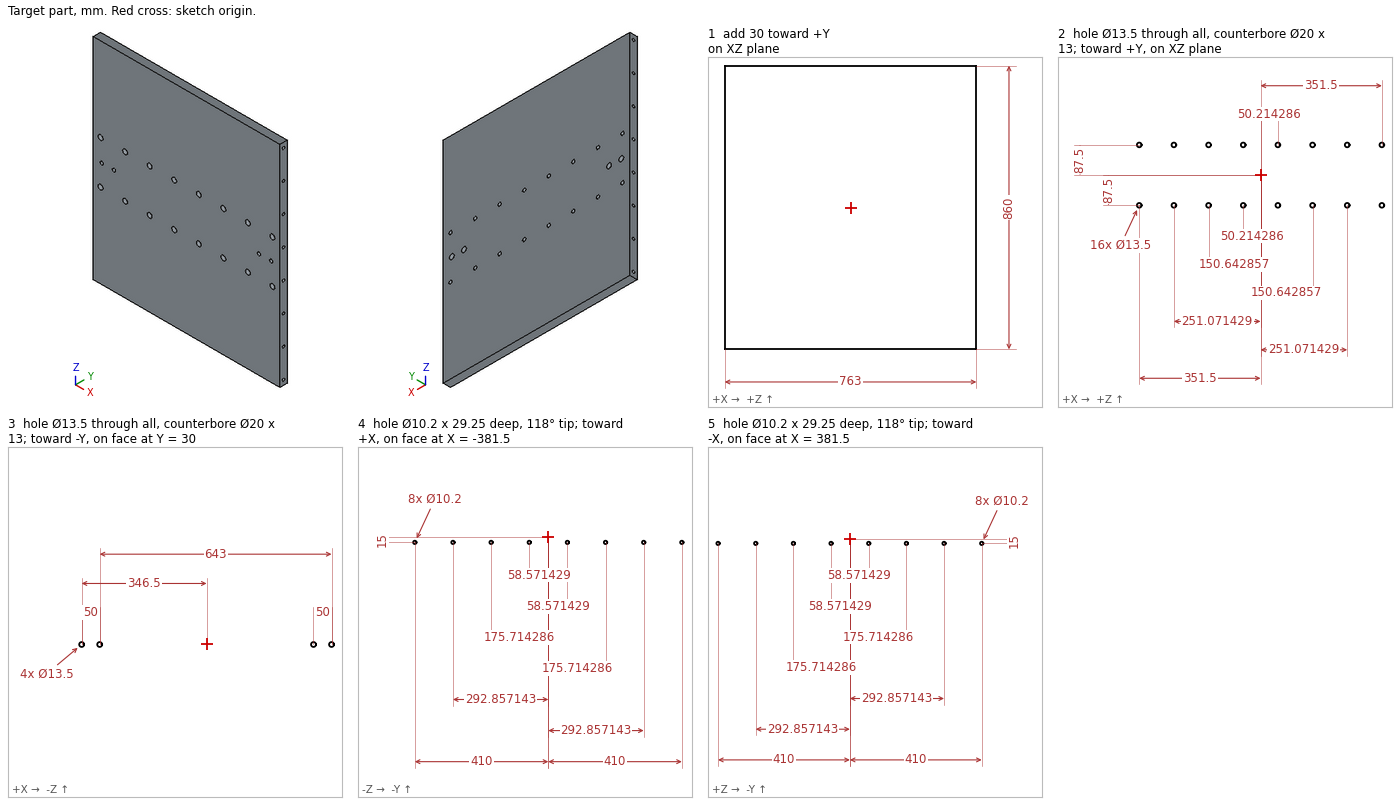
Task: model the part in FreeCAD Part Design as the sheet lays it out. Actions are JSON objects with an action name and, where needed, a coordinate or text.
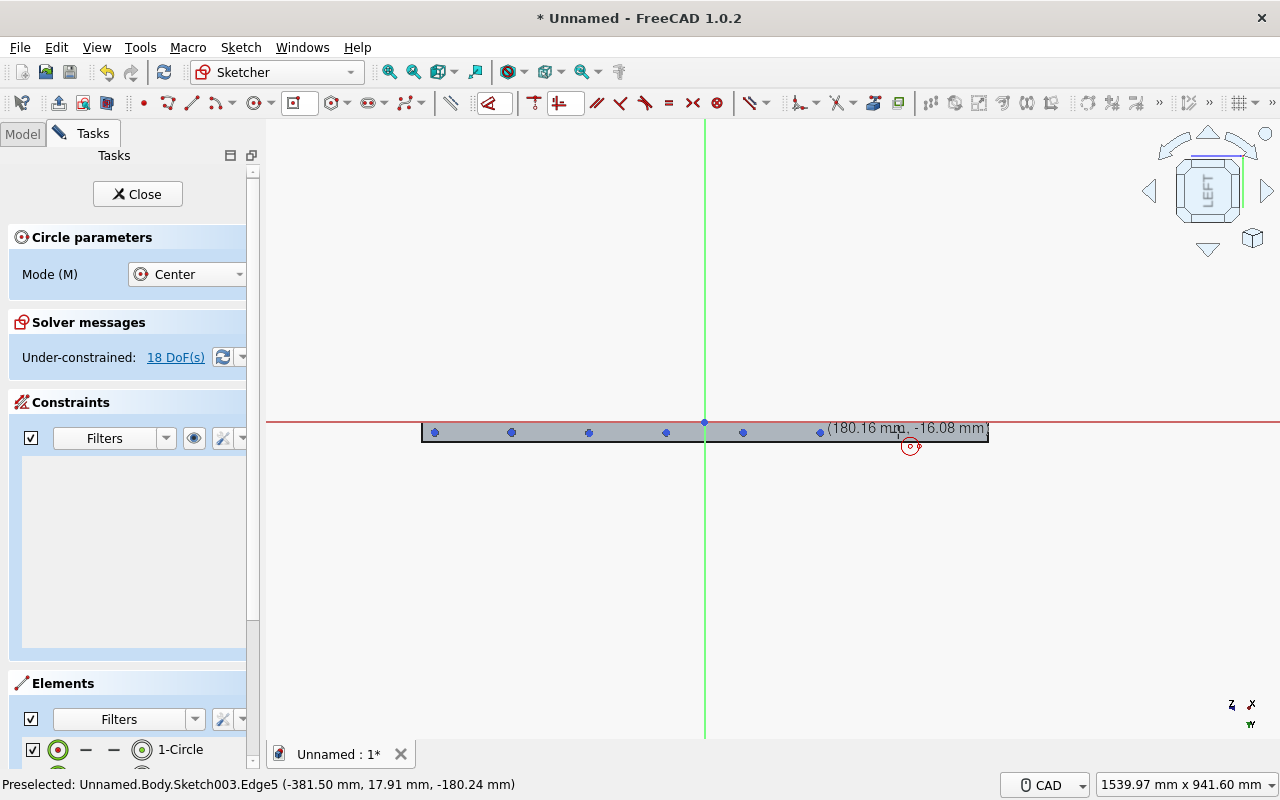
{"action": "scroll", "coordinate": [898, 432], "scroll_direction": "up", "scroll_amount": 3}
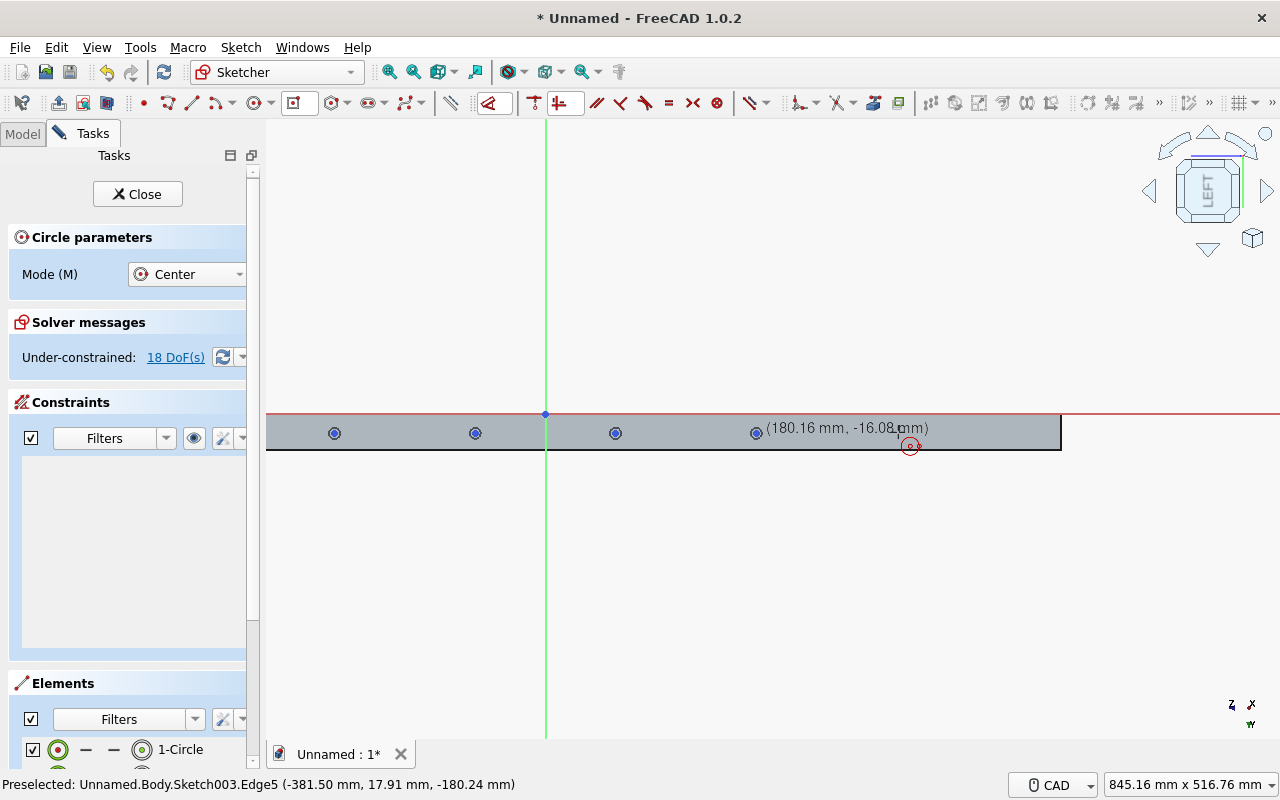
{"action": "left_click", "coordinate": [897, 432]}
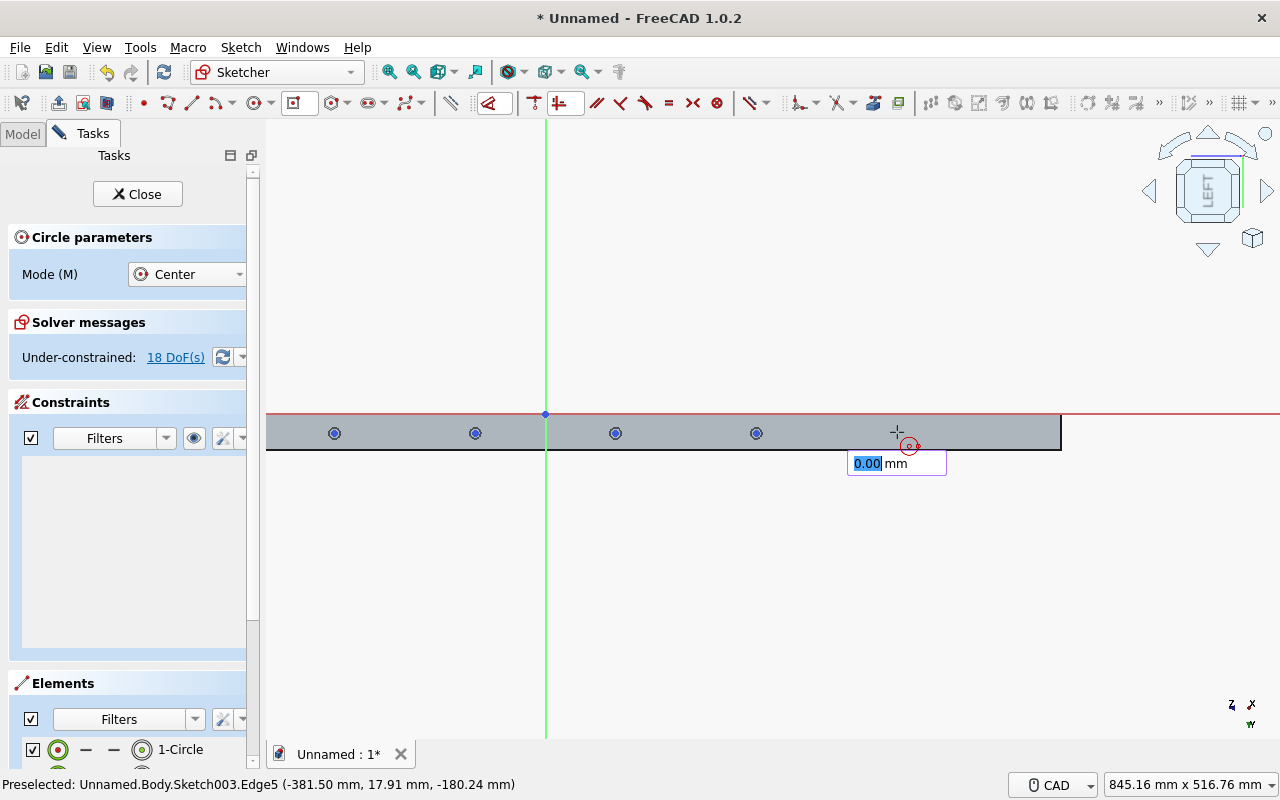
{"action": "scroll", "coordinate": [901, 436], "scroll_direction": "up", "scroll_amount": 5}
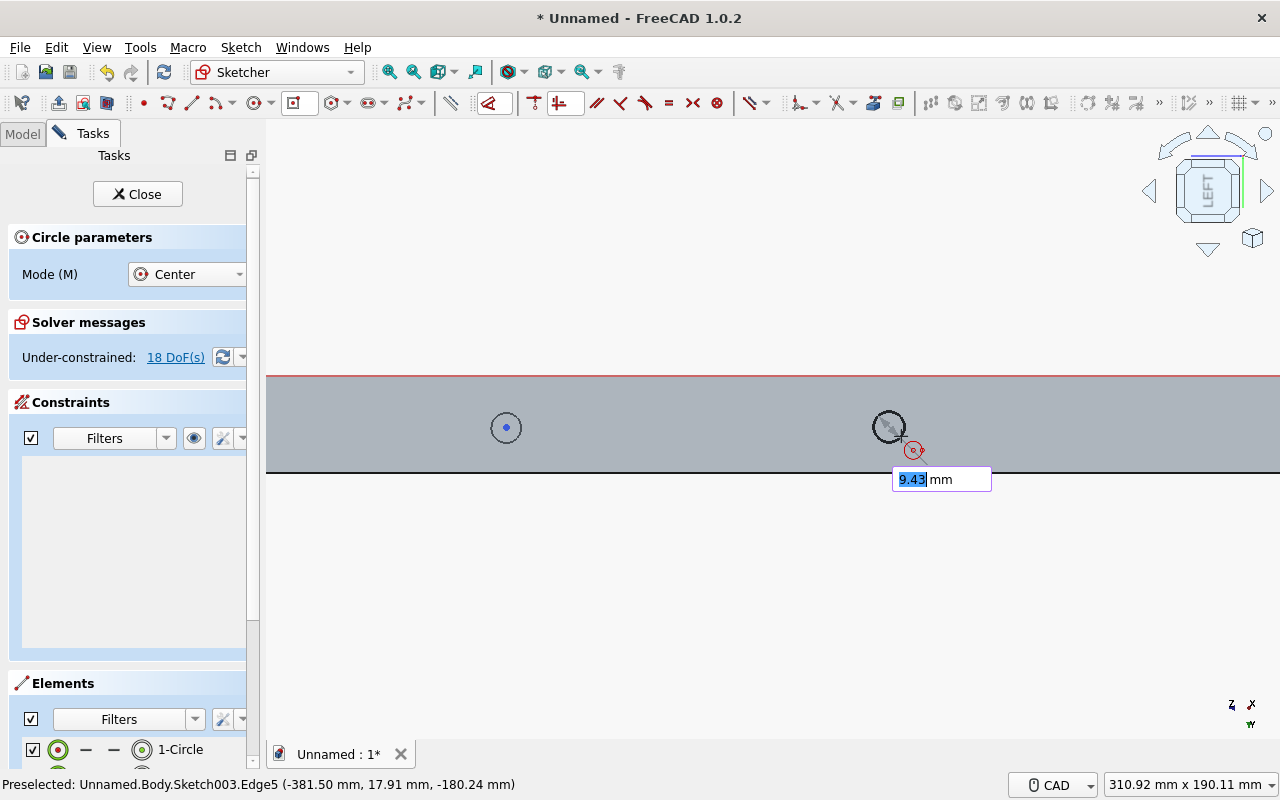
{"action": "left_click", "coordinate": [900, 436]}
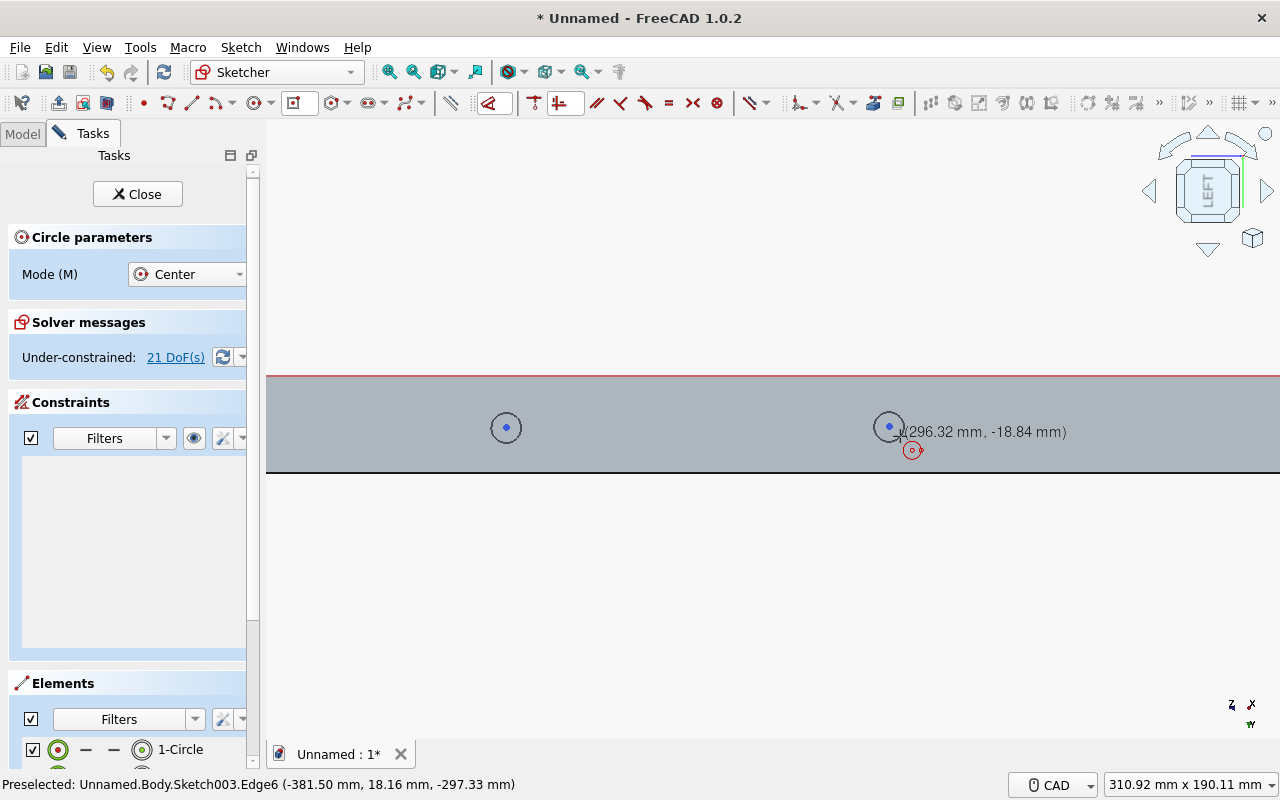
{"action": "scroll", "coordinate": [900, 434], "scroll_direction": "down", "scroll_amount": 8}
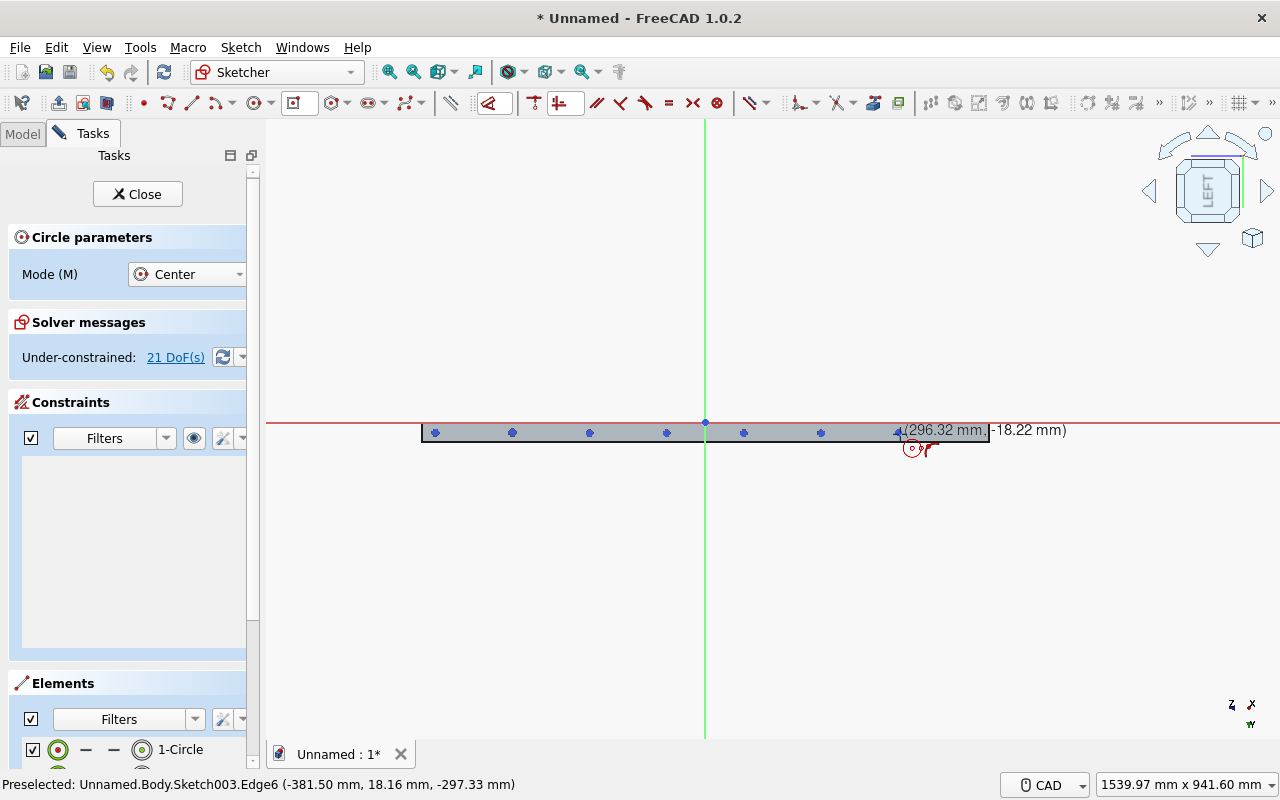
{"action": "scroll", "coordinate": [975, 432], "scroll_direction": "up", "scroll_amount": 10}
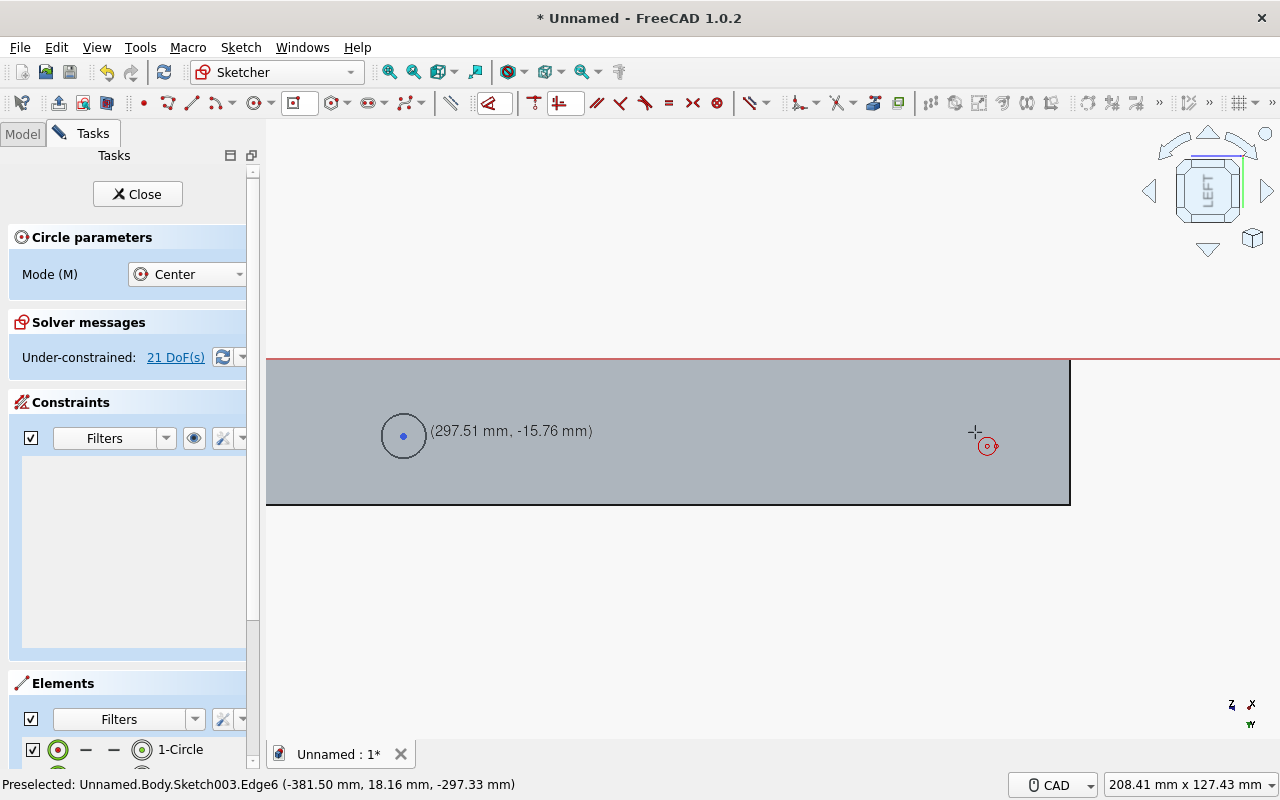
{"action": "scroll", "coordinate": [975, 432], "scroll_direction": "down", "scroll_amount": 10}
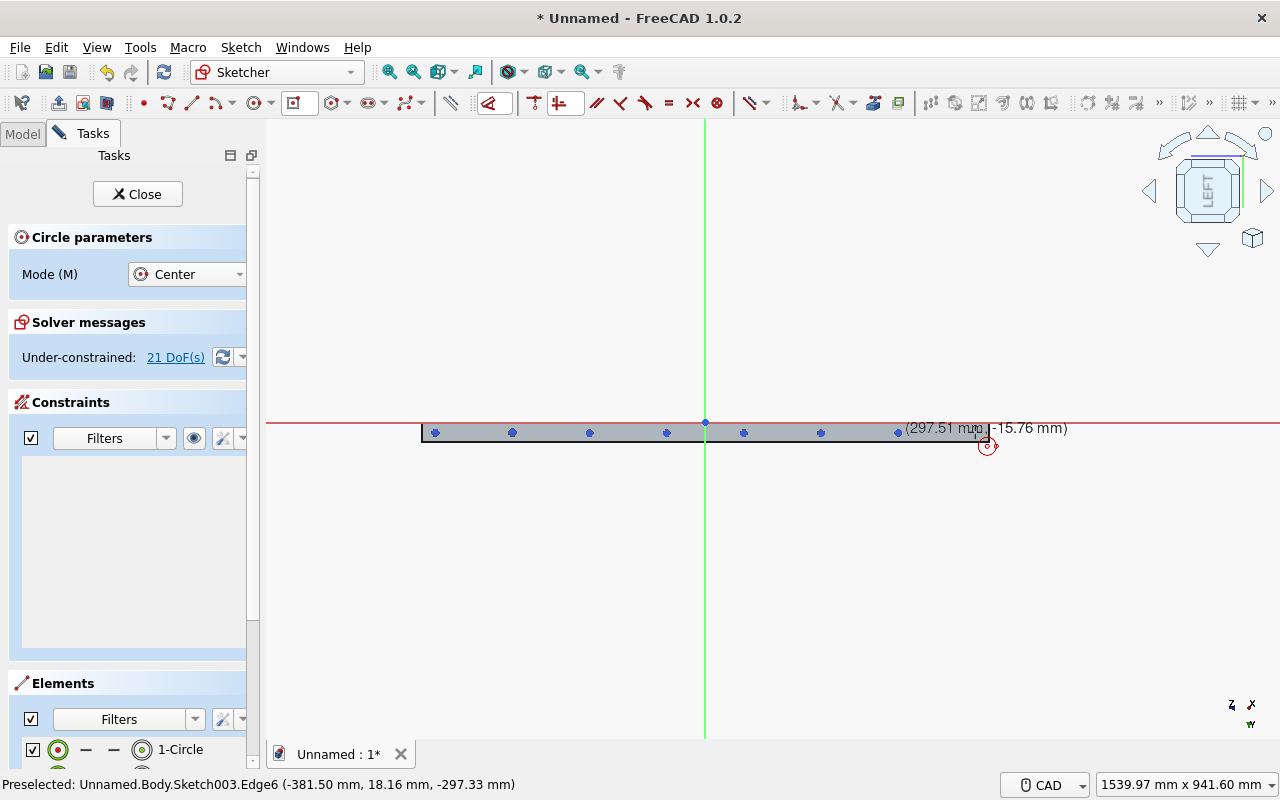
{"action": "scroll", "coordinate": [975, 432], "scroll_direction": "up", "scroll_amount": 3}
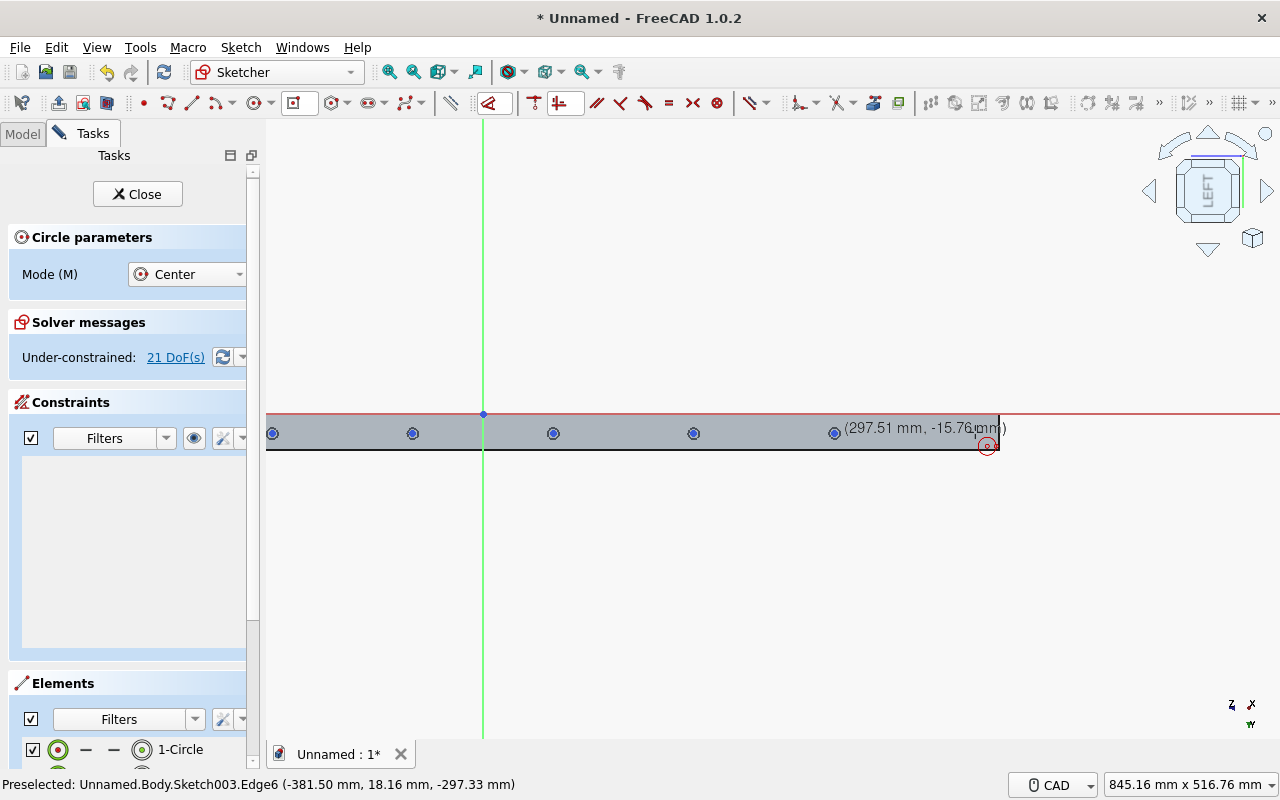
{"action": "left_click", "coordinate": [975, 432]}